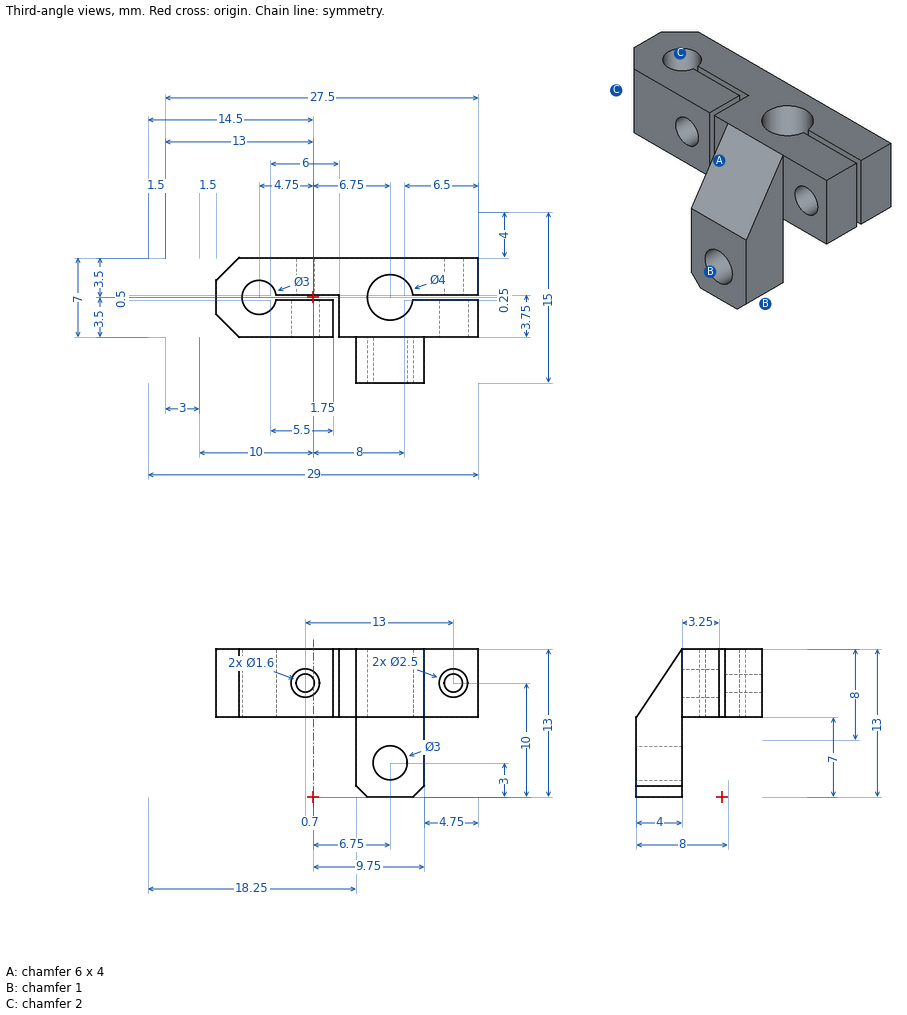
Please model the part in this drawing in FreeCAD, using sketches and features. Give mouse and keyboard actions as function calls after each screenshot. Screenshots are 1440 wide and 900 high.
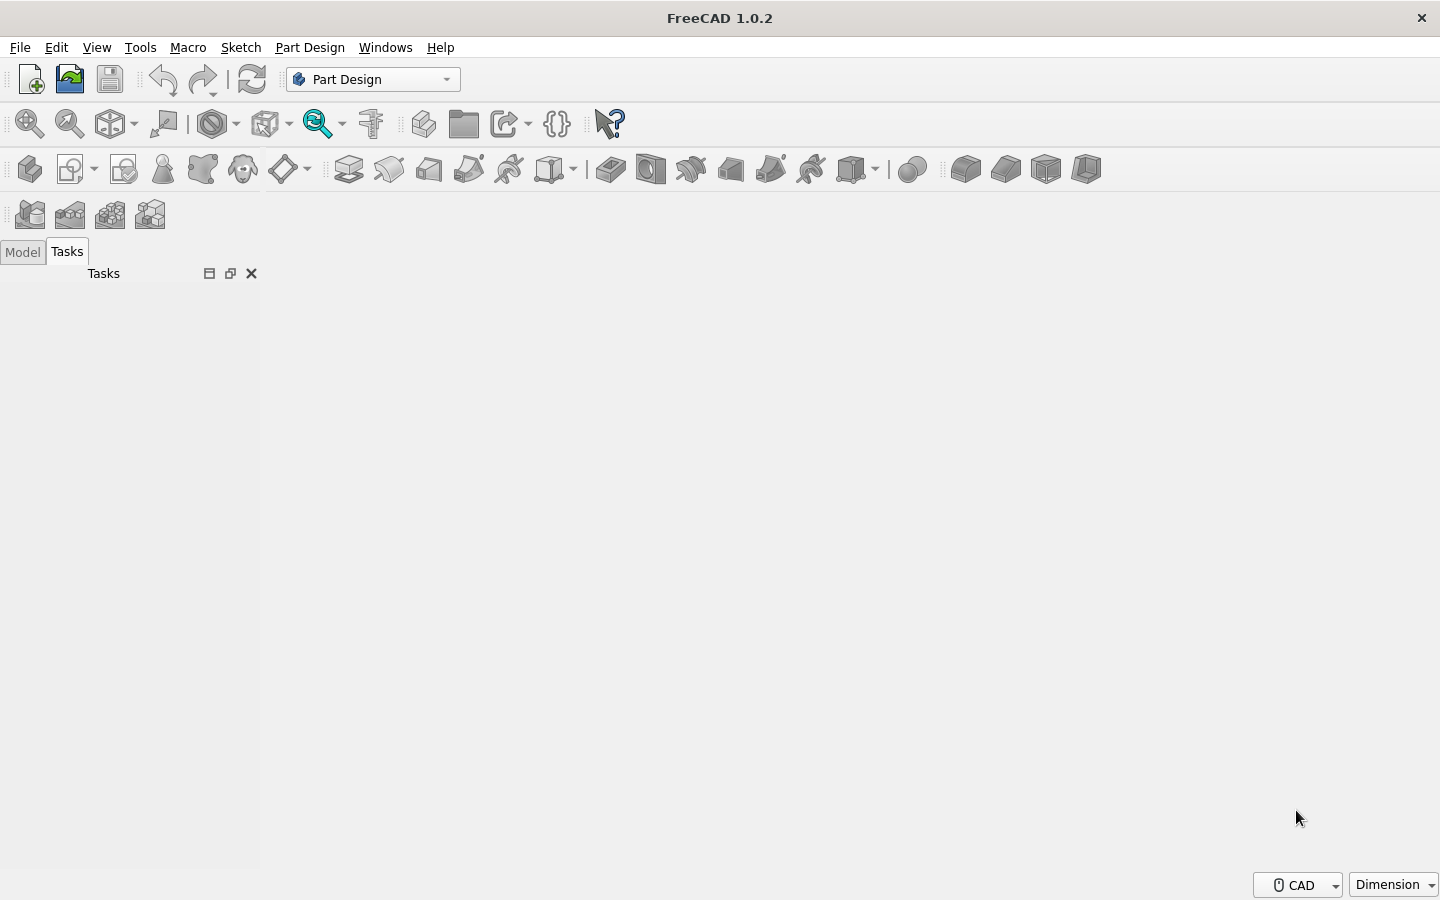
click(30, 80)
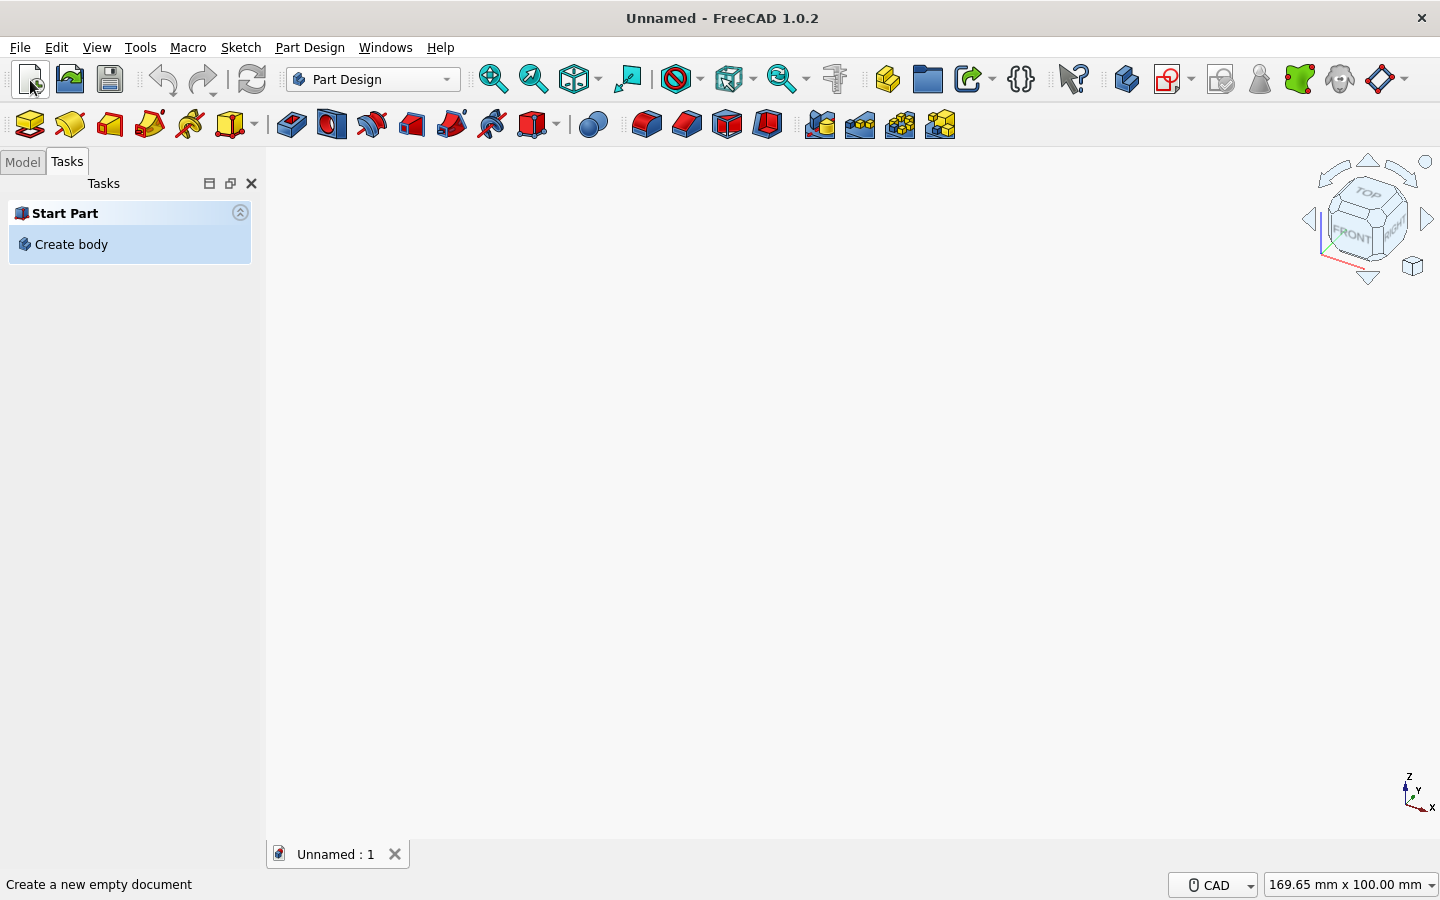
click(1168, 80)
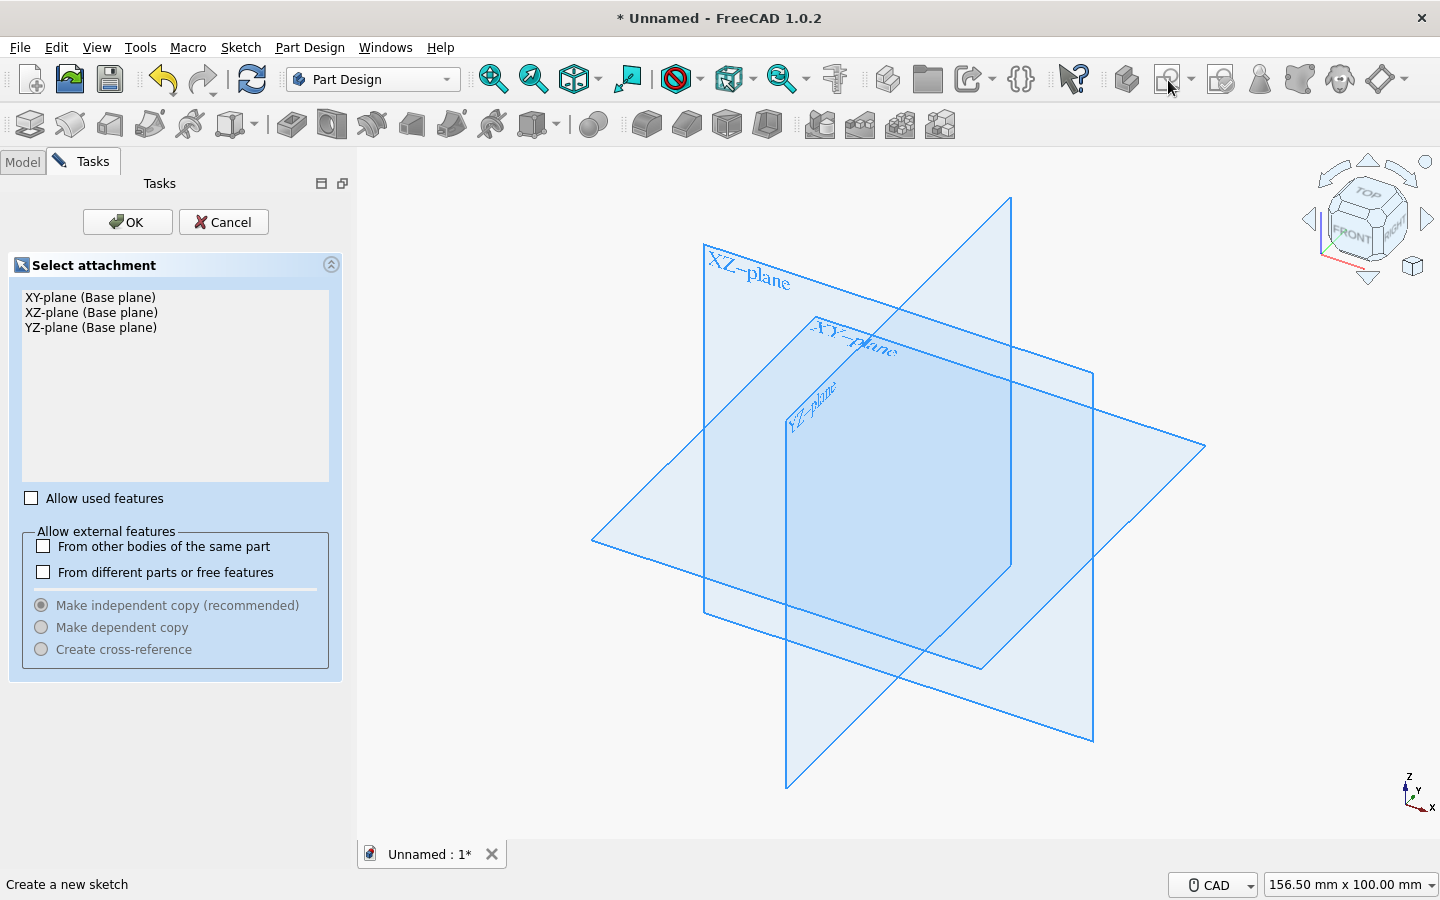
click(82, 298)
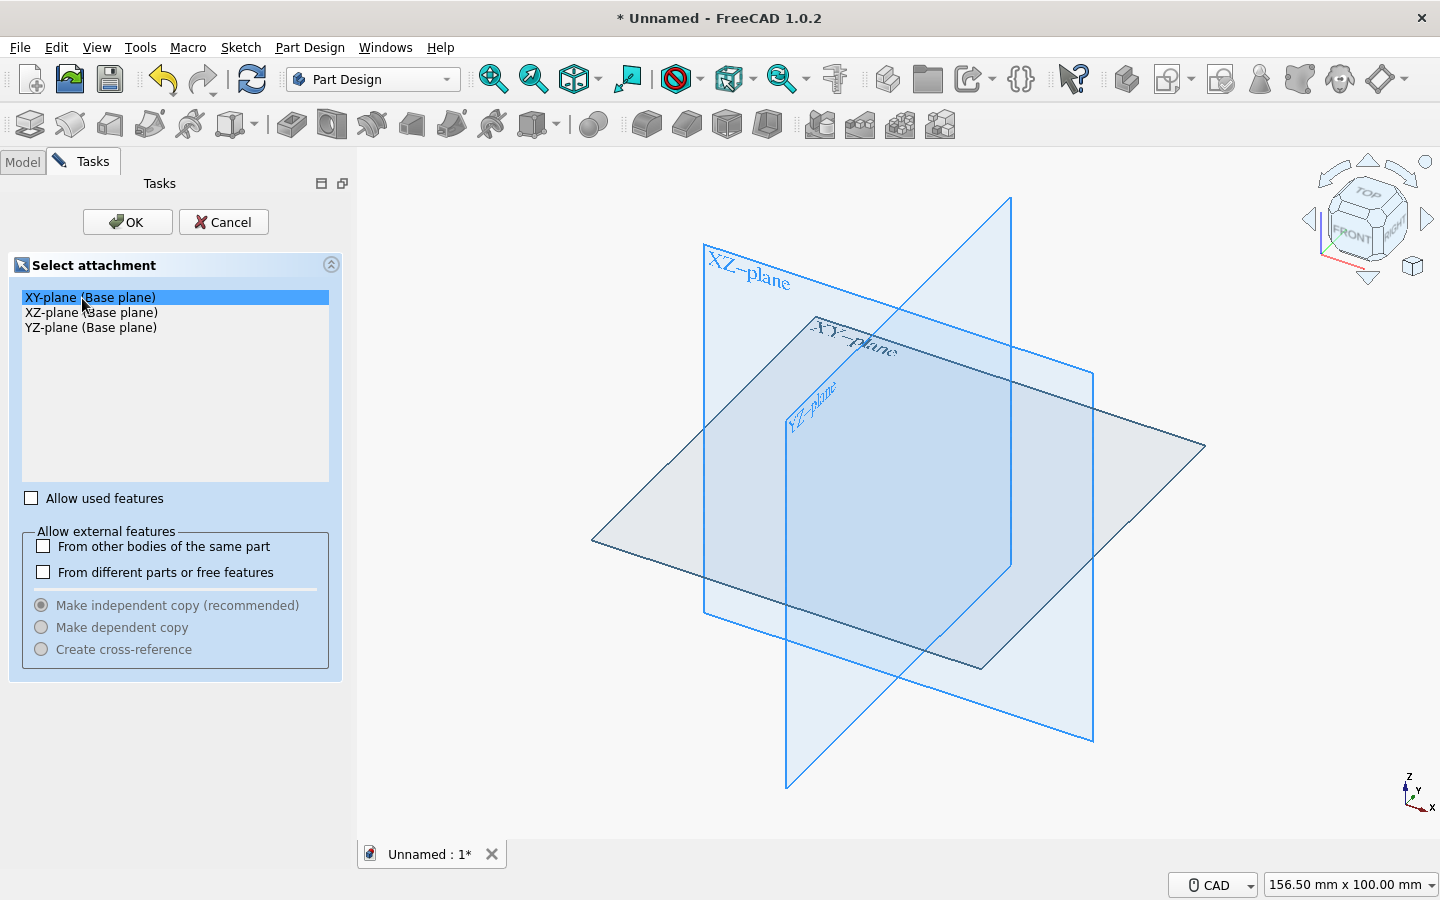
click(128, 222)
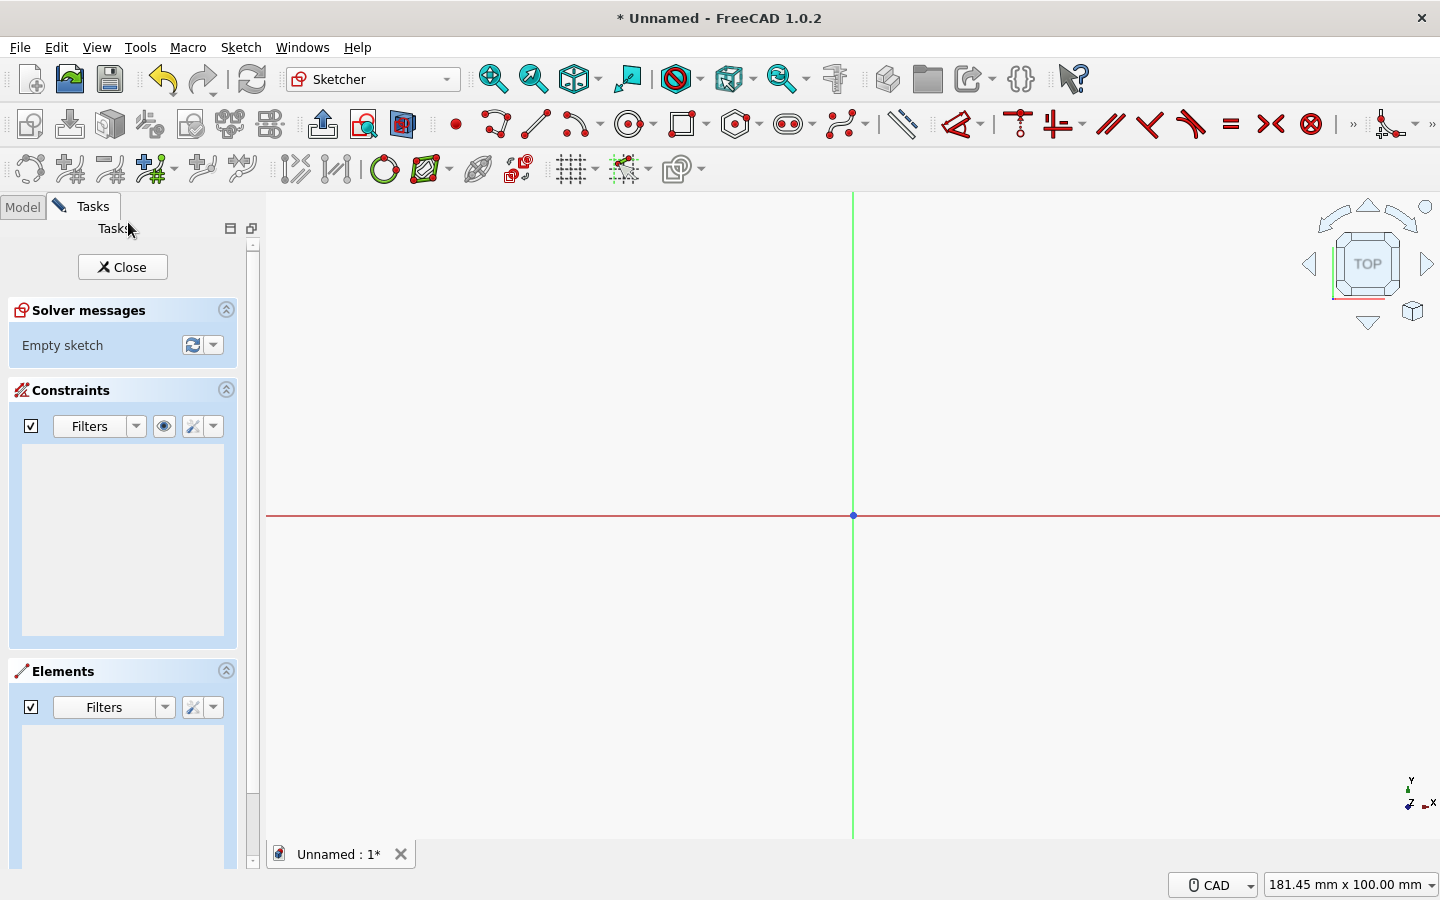
scroll(875, 516, up, 7)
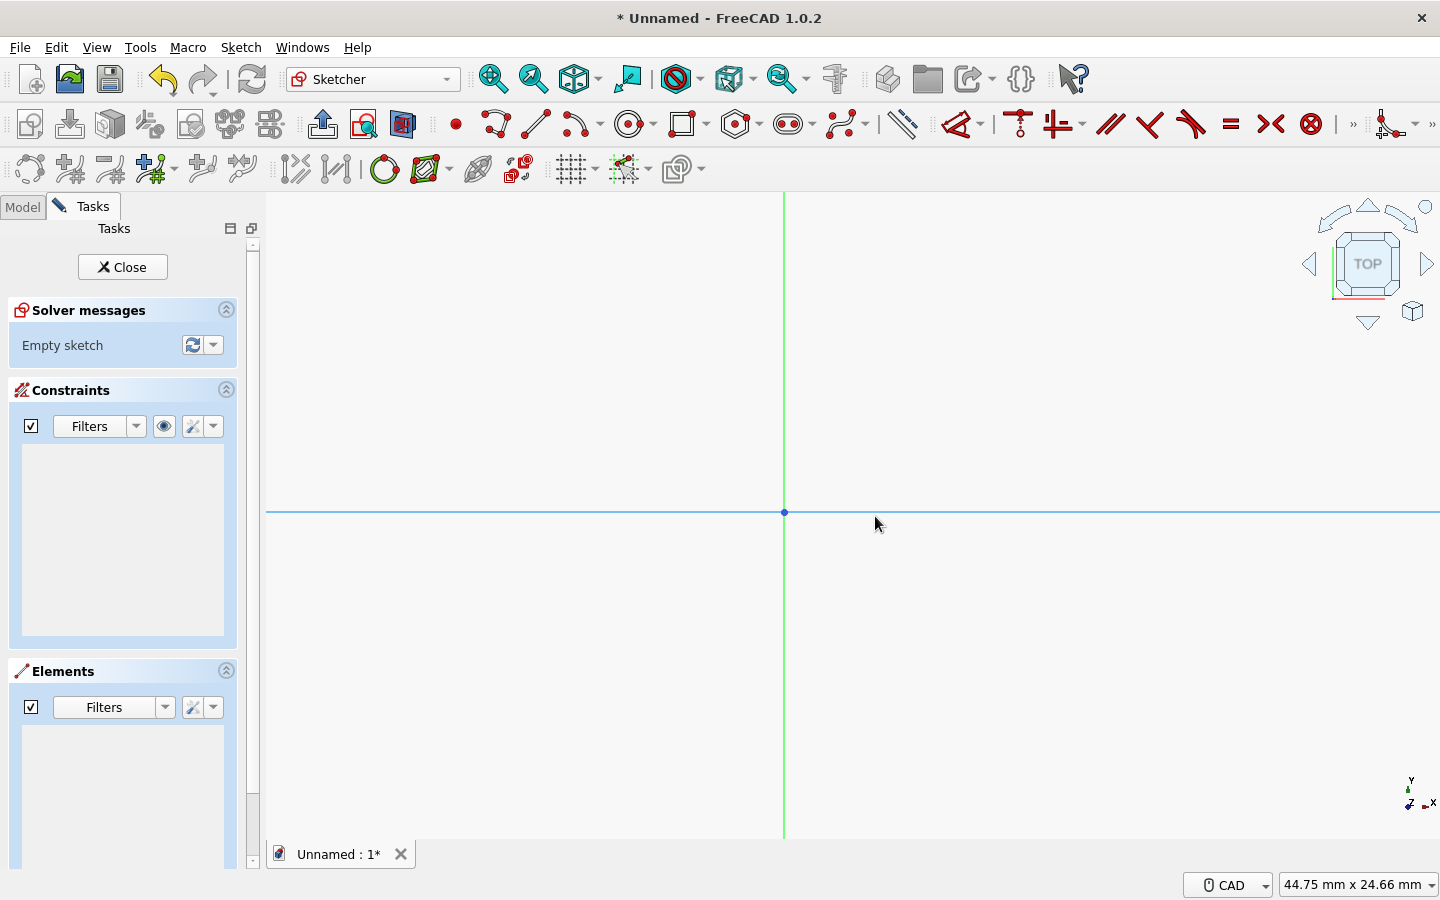
click(708, 124)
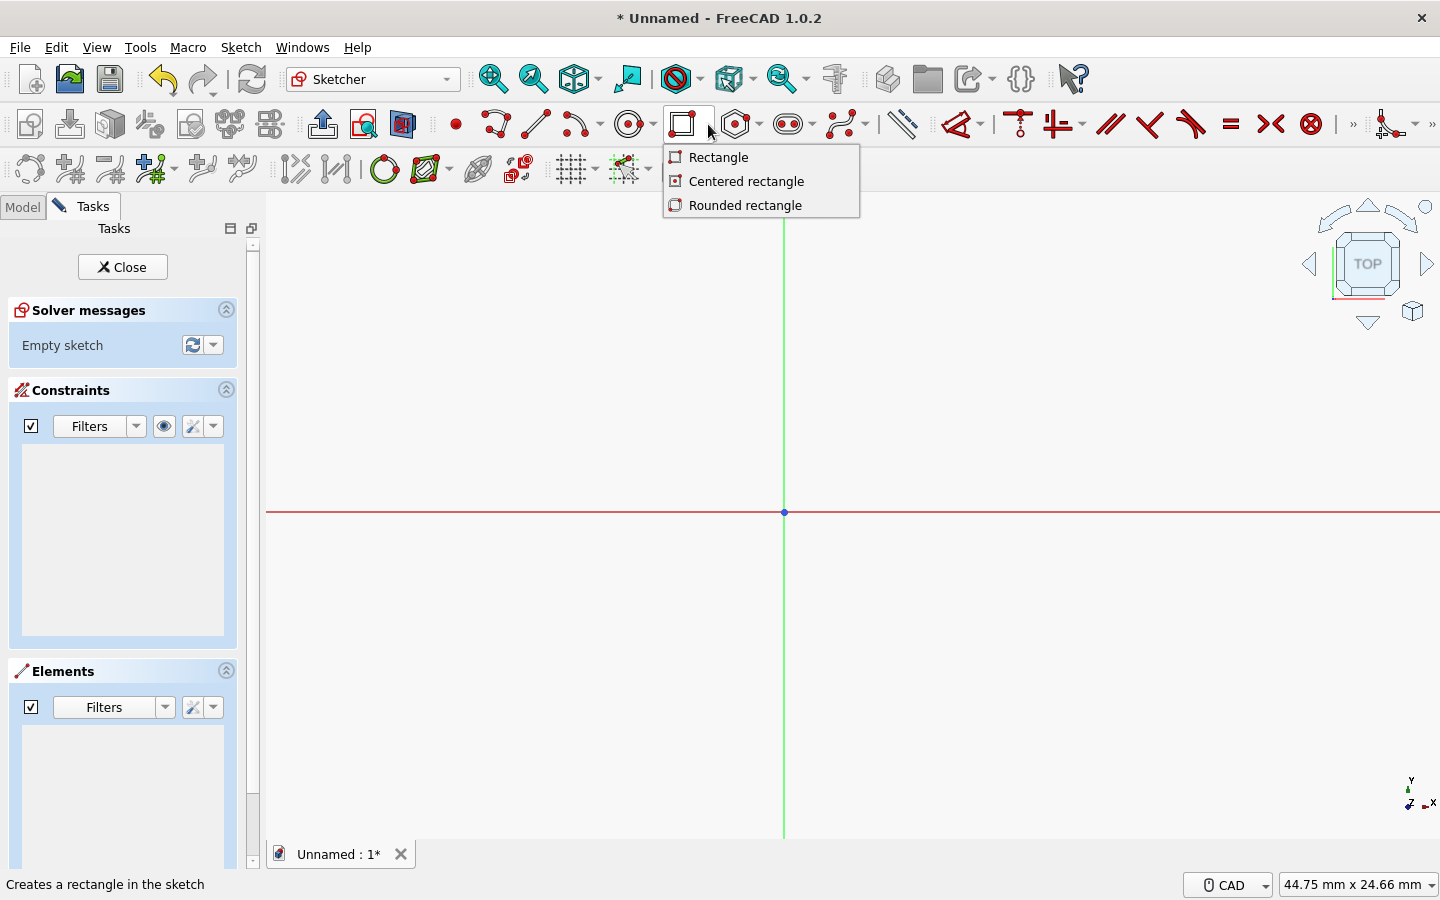
click(762, 181)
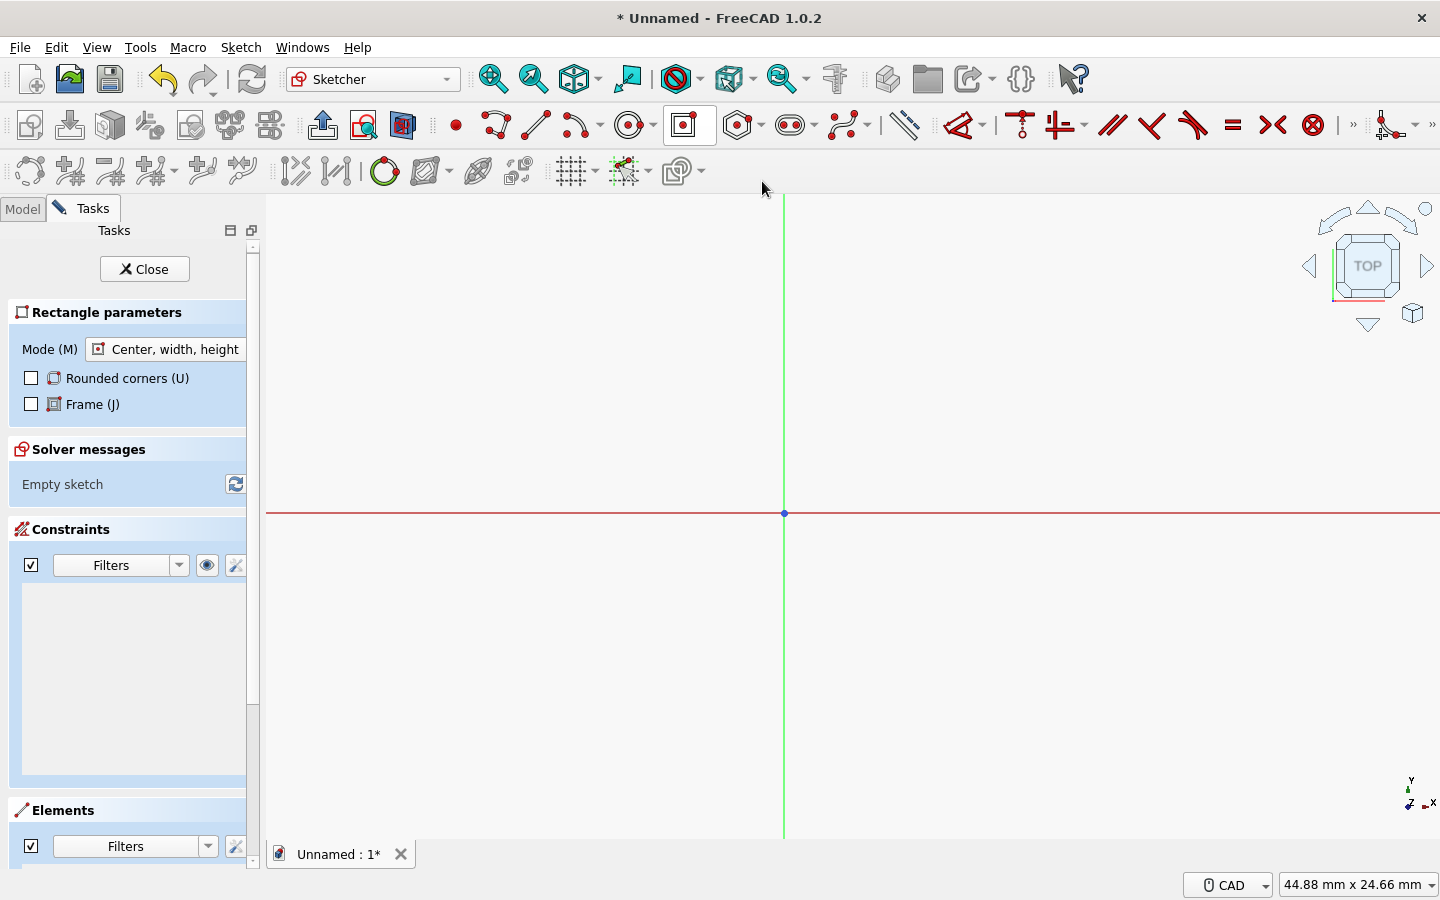
click(784, 513)
move(1164, 317)